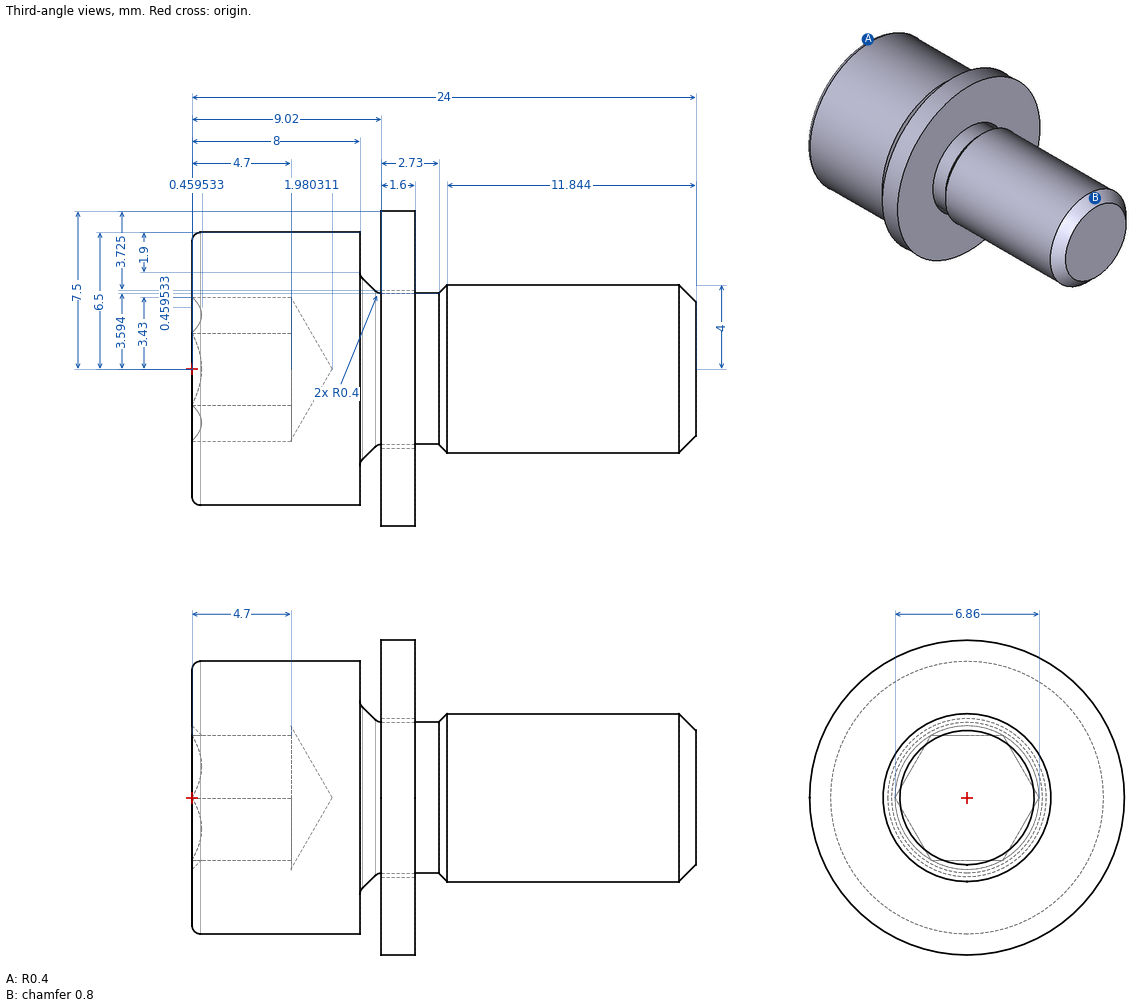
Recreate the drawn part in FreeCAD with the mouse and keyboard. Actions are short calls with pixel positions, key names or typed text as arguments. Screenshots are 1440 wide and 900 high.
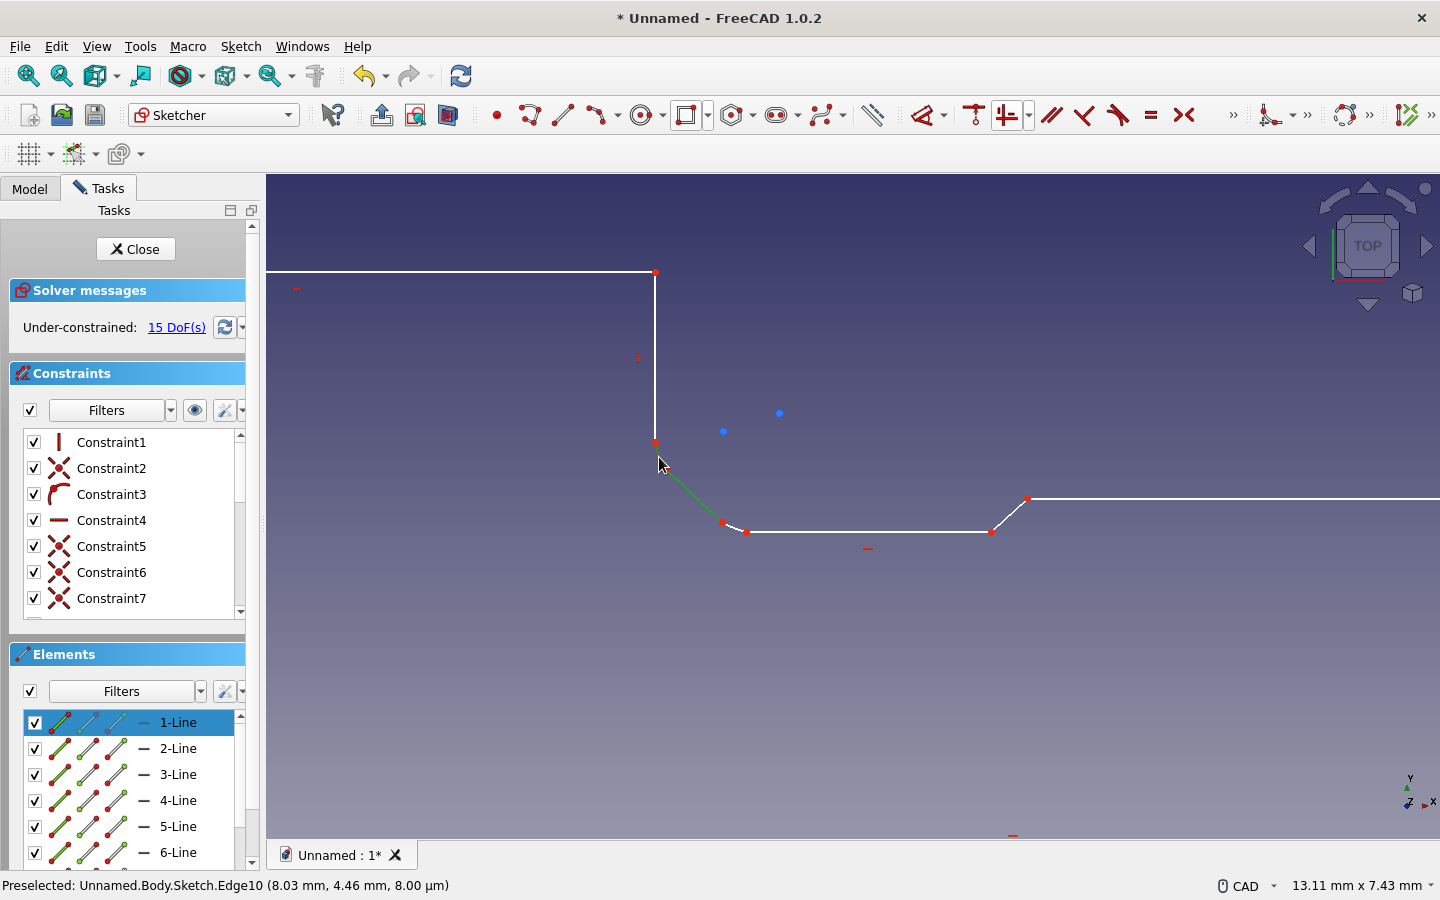
click(1118, 116)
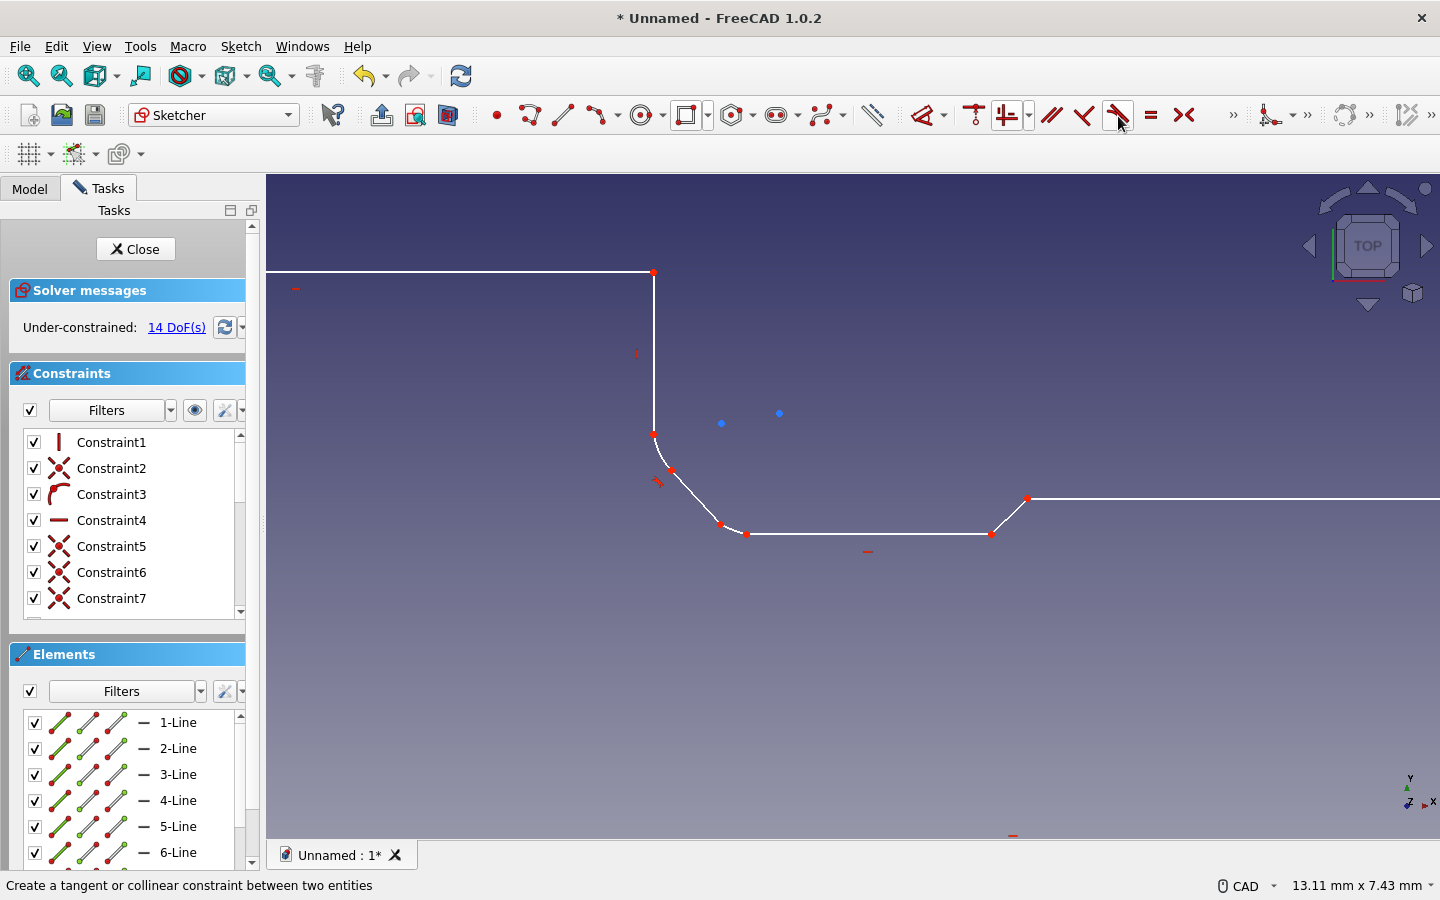
click(706, 508)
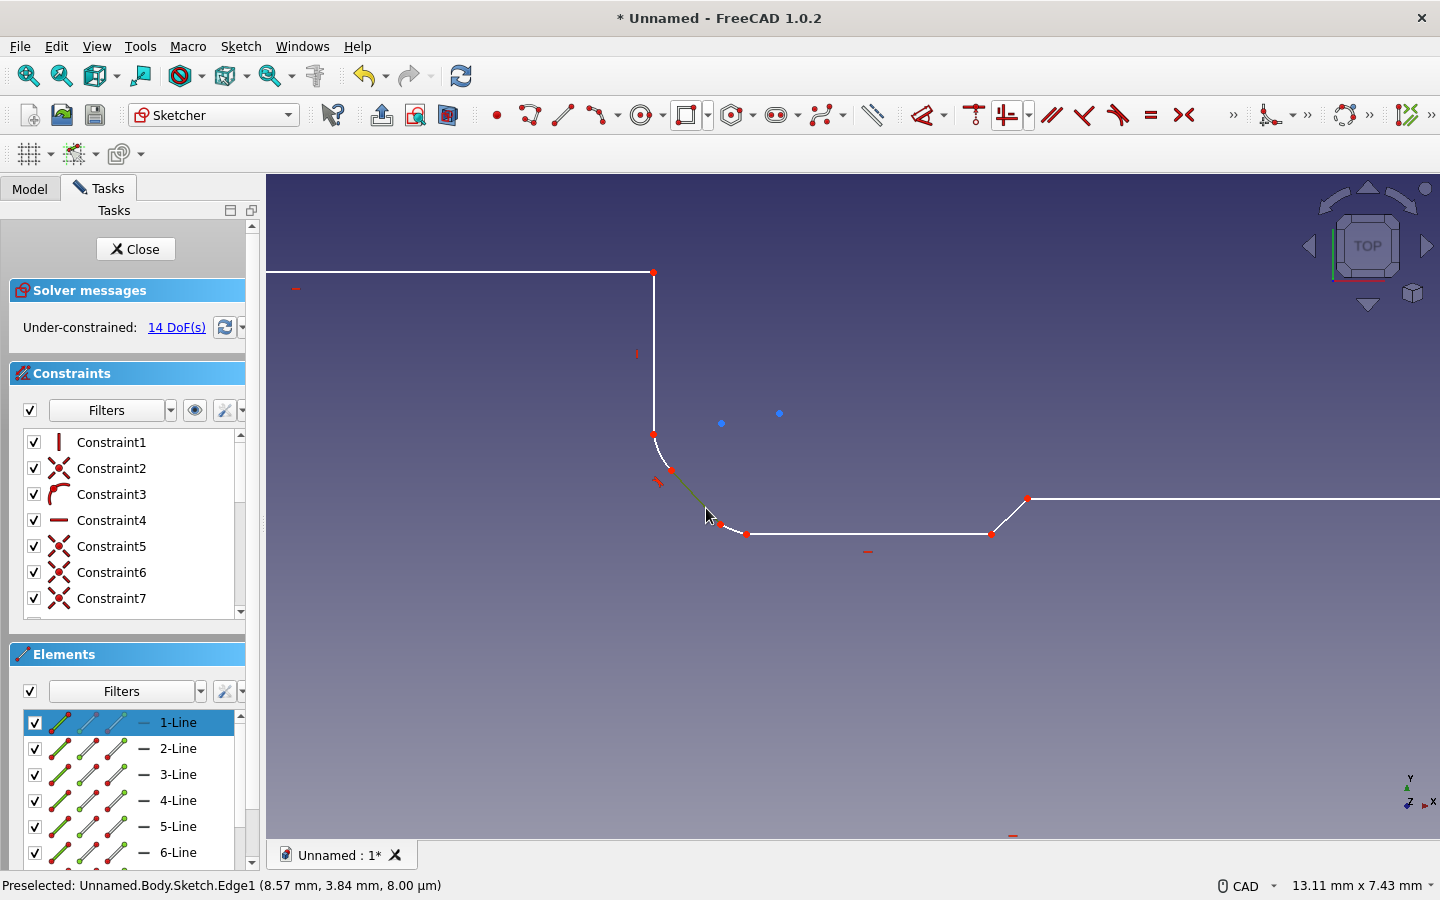
click(733, 530)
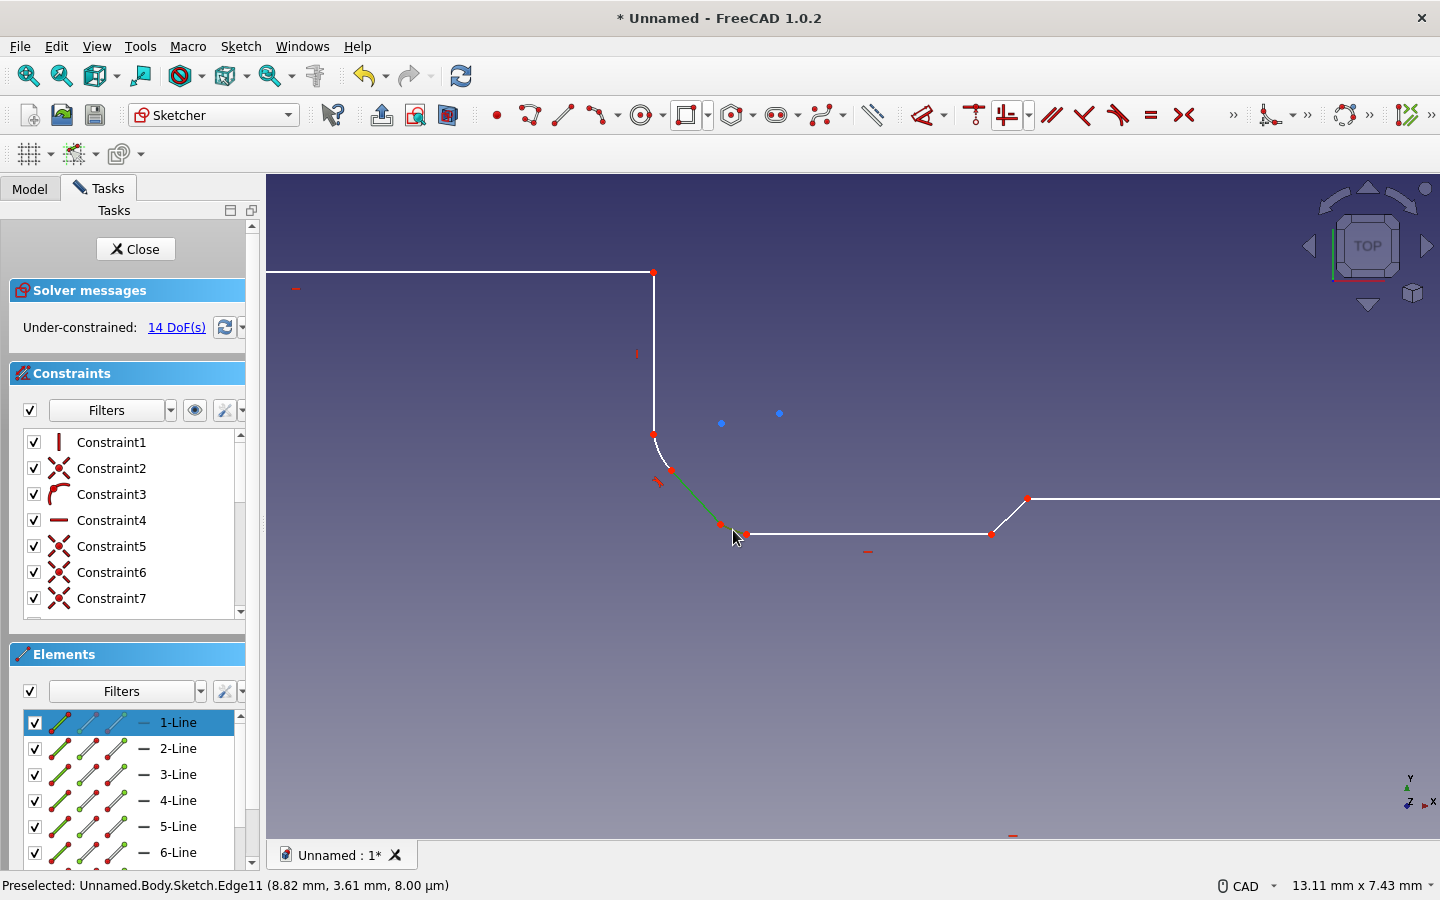
click(1118, 116)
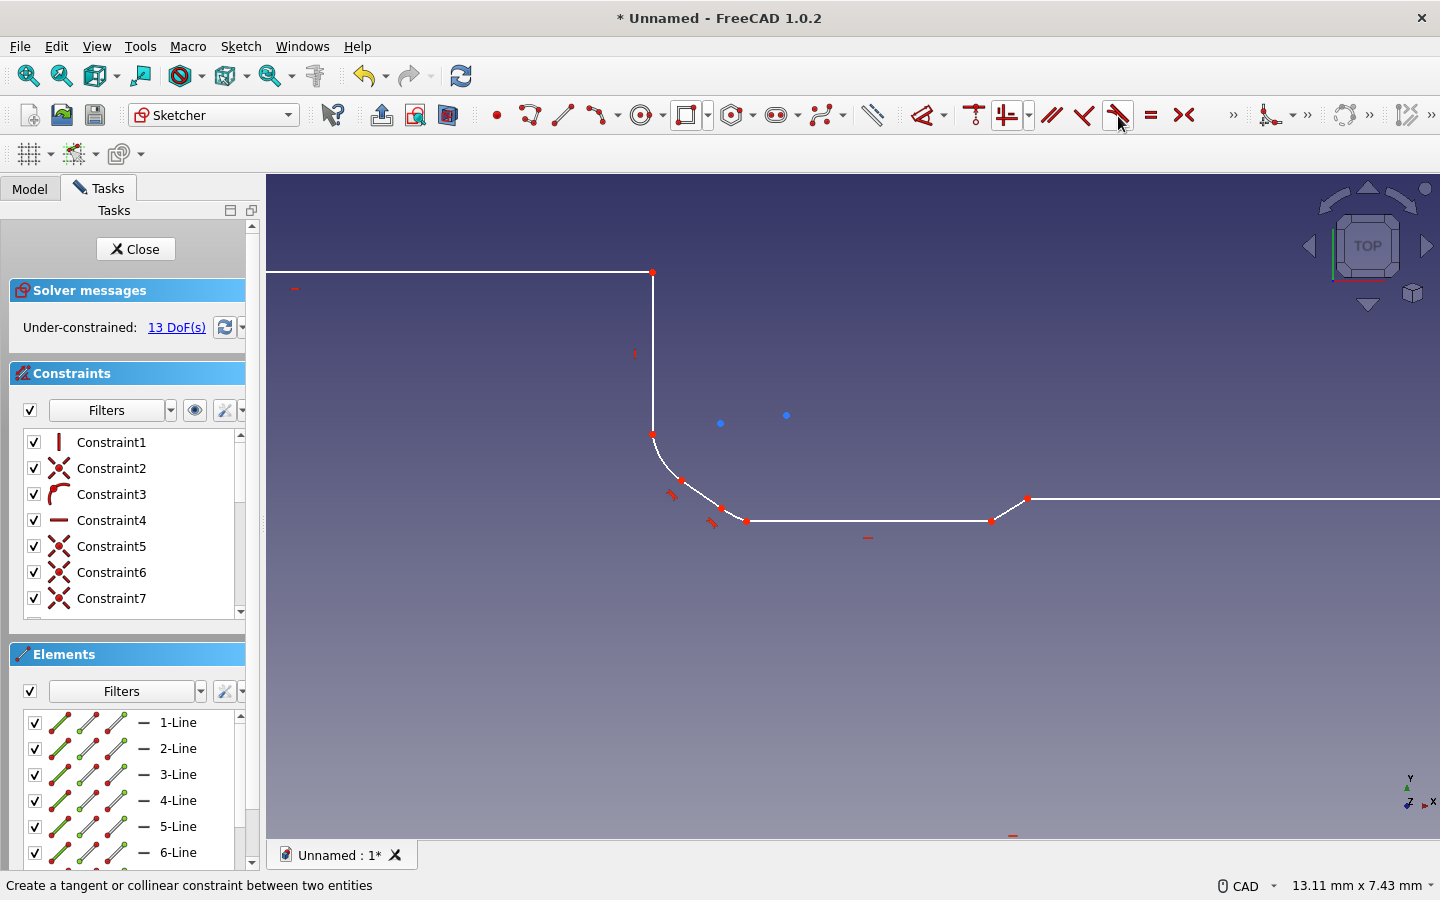
click(653, 386)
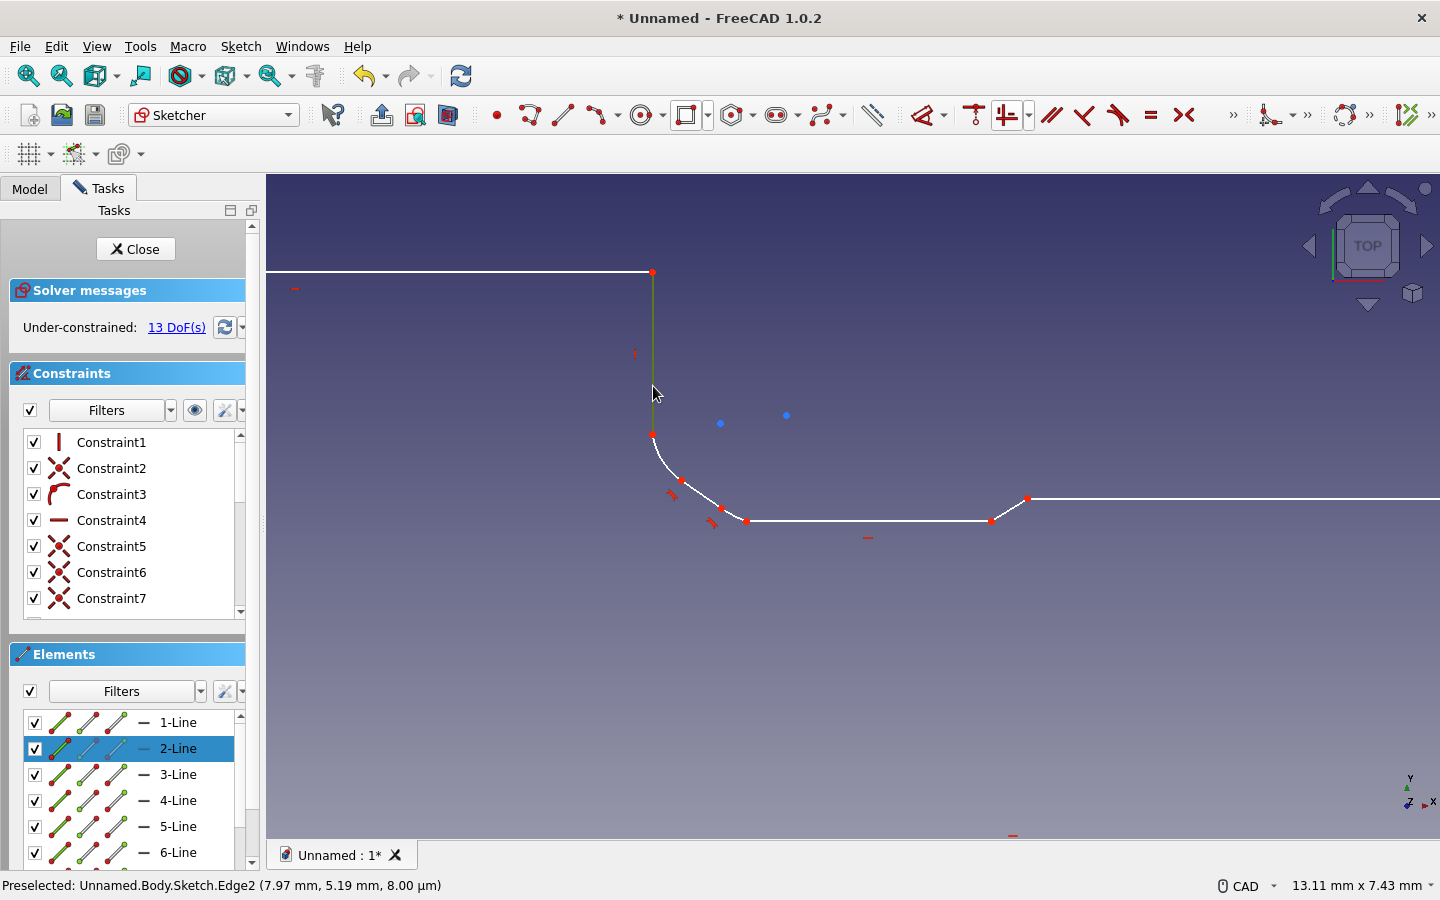
click(657, 451)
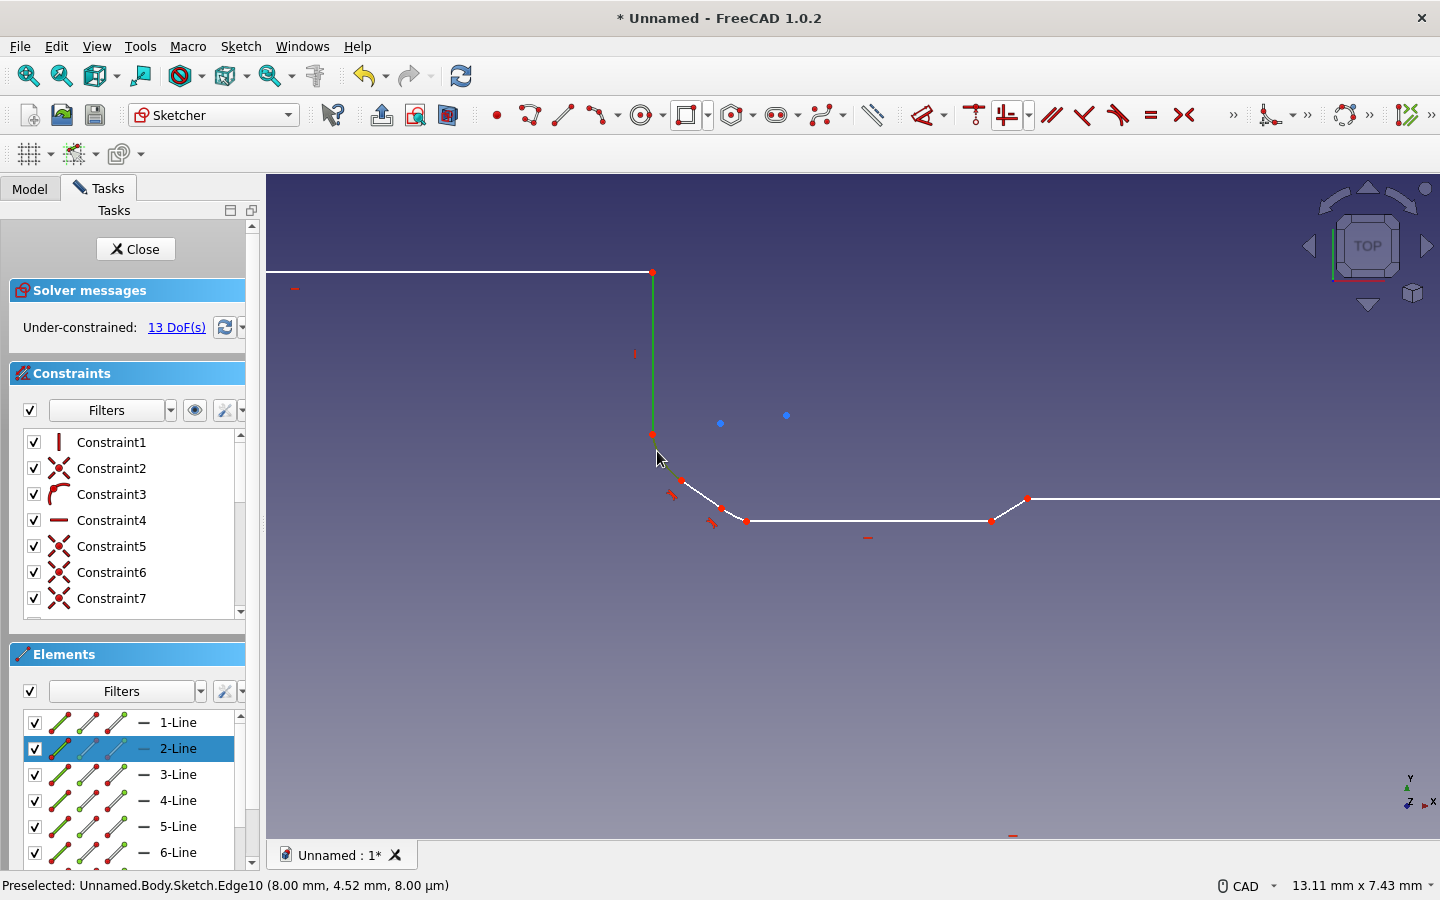
click(1118, 116)